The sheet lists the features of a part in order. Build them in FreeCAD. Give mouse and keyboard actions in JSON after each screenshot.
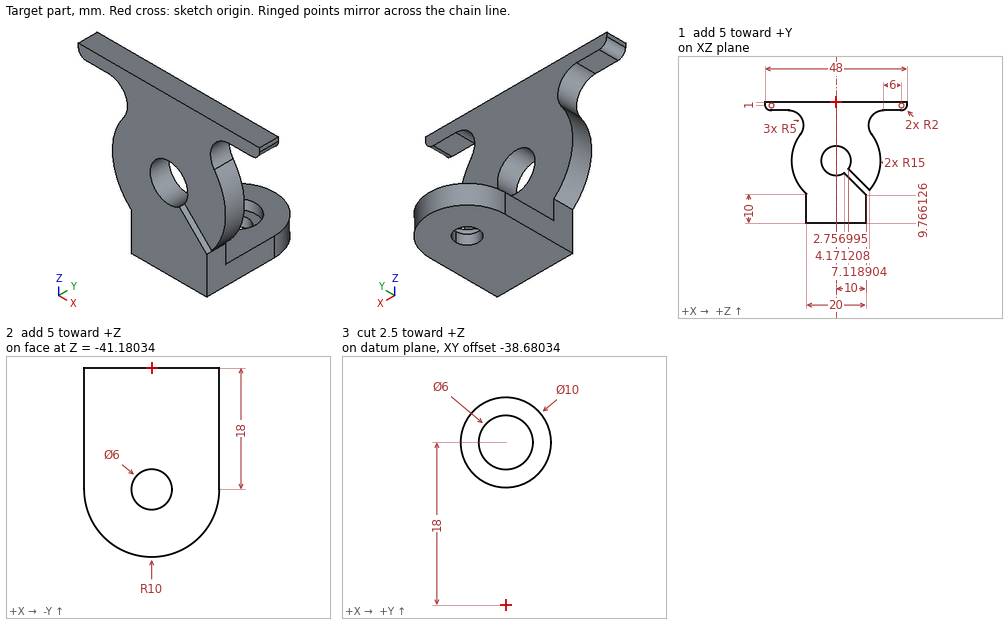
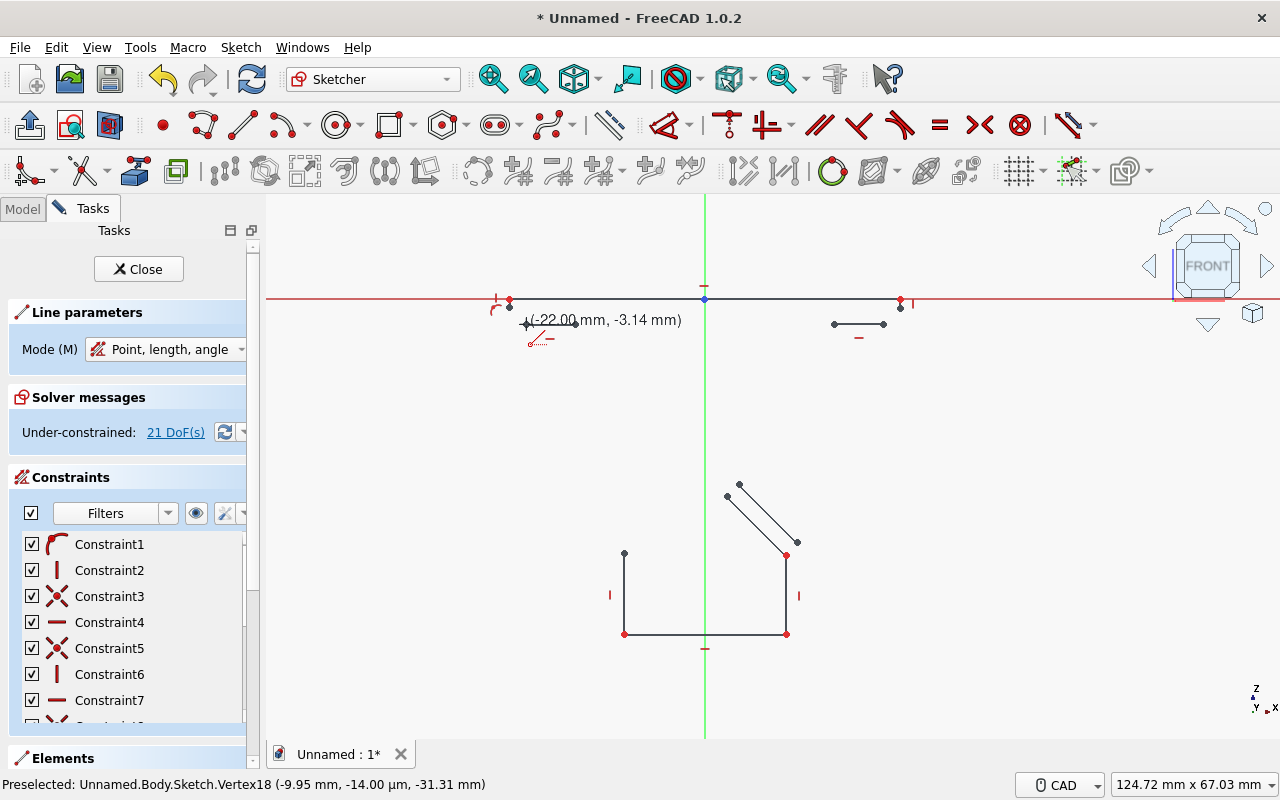
{"action": "key", "text": "g 3 a"}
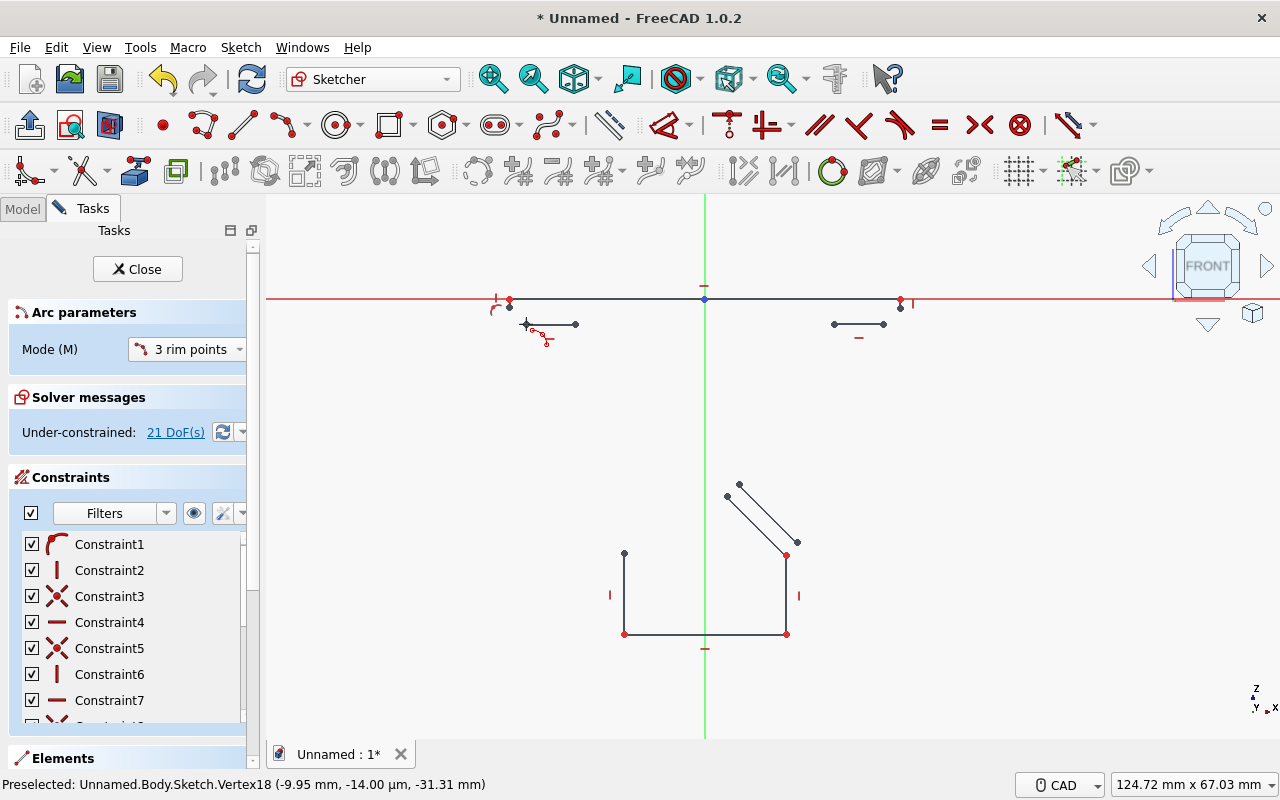
{"action": "scroll", "coordinate": [900, 308], "scroll_direction": "up", "scroll_amount": 7}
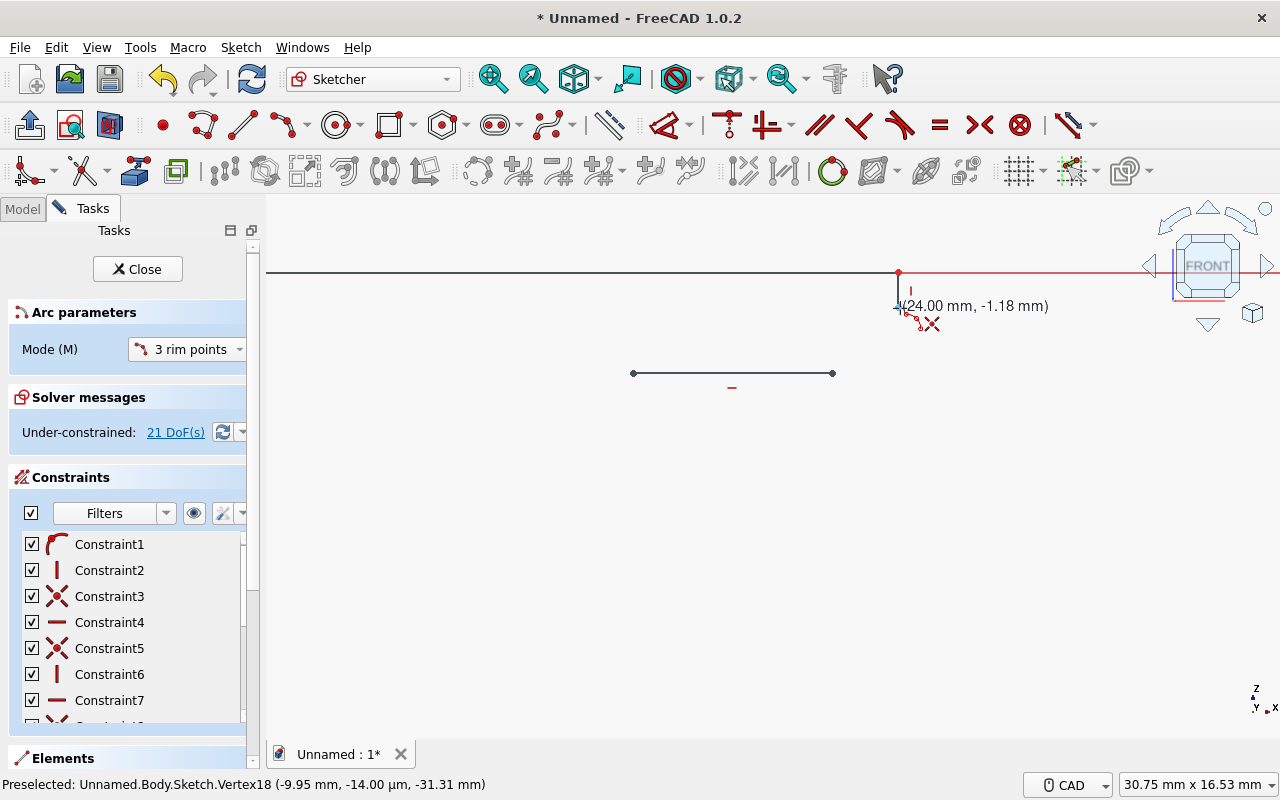
{"action": "left_click", "coordinate": [898, 308]}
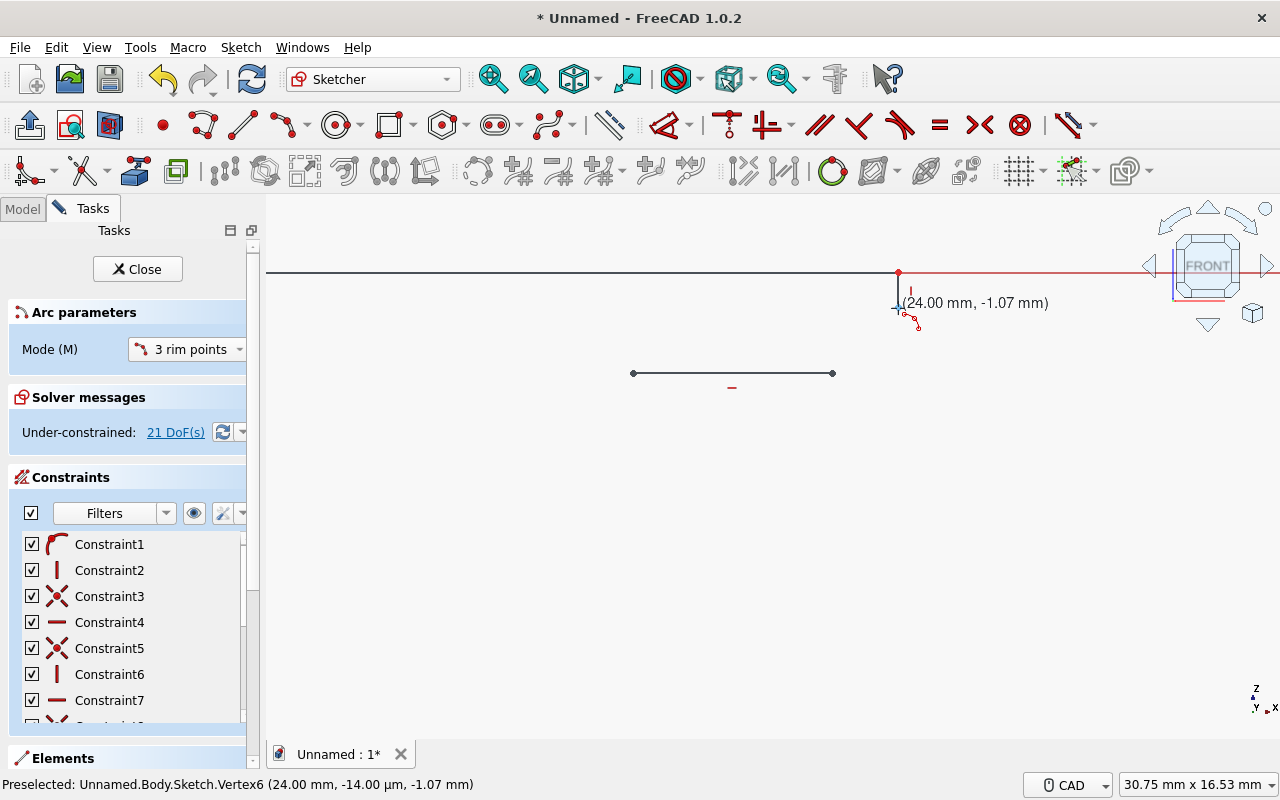
{"action": "scroll", "coordinate": [900, 308], "scroll_direction": "down", "scroll_amount": 7}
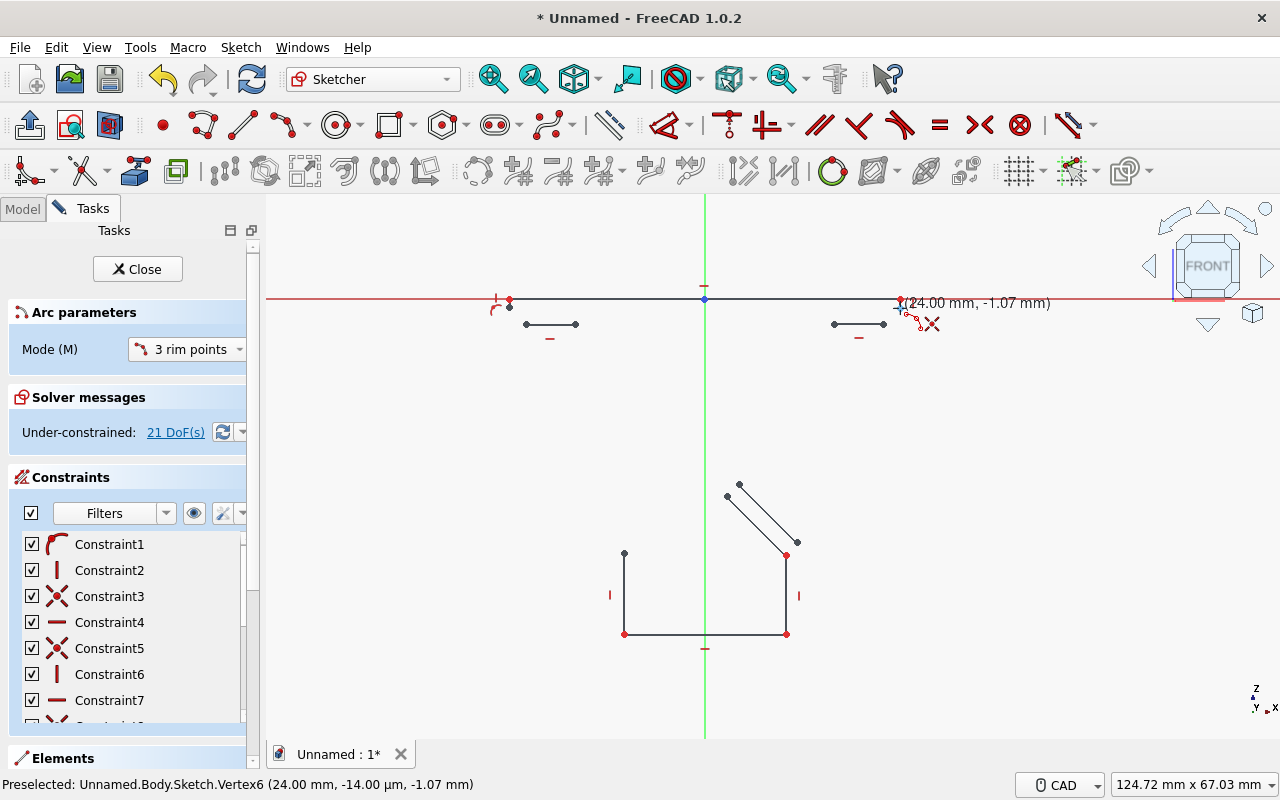
{"action": "left_click", "coordinate": [884, 324]}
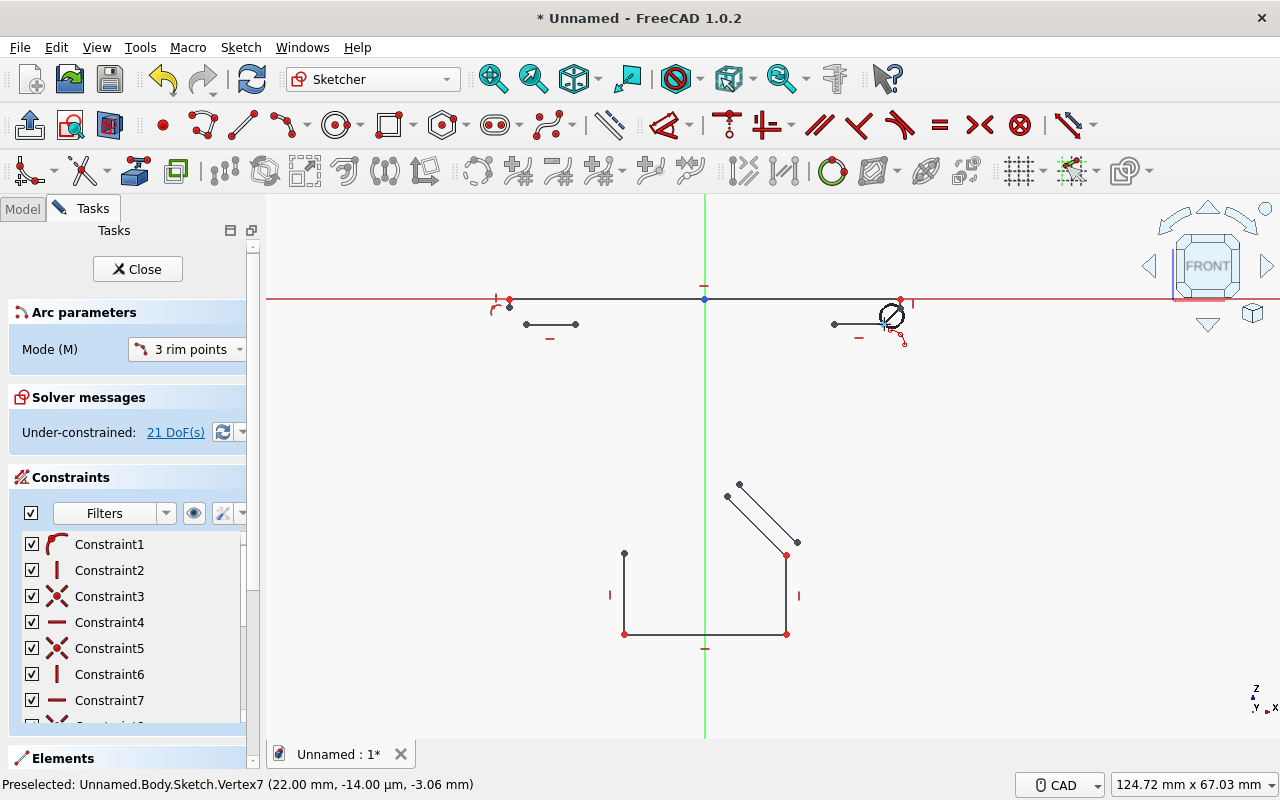
{"action": "scroll", "coordinate": [895, 319], "scroll_direction": "up", "scroll_amount": 7}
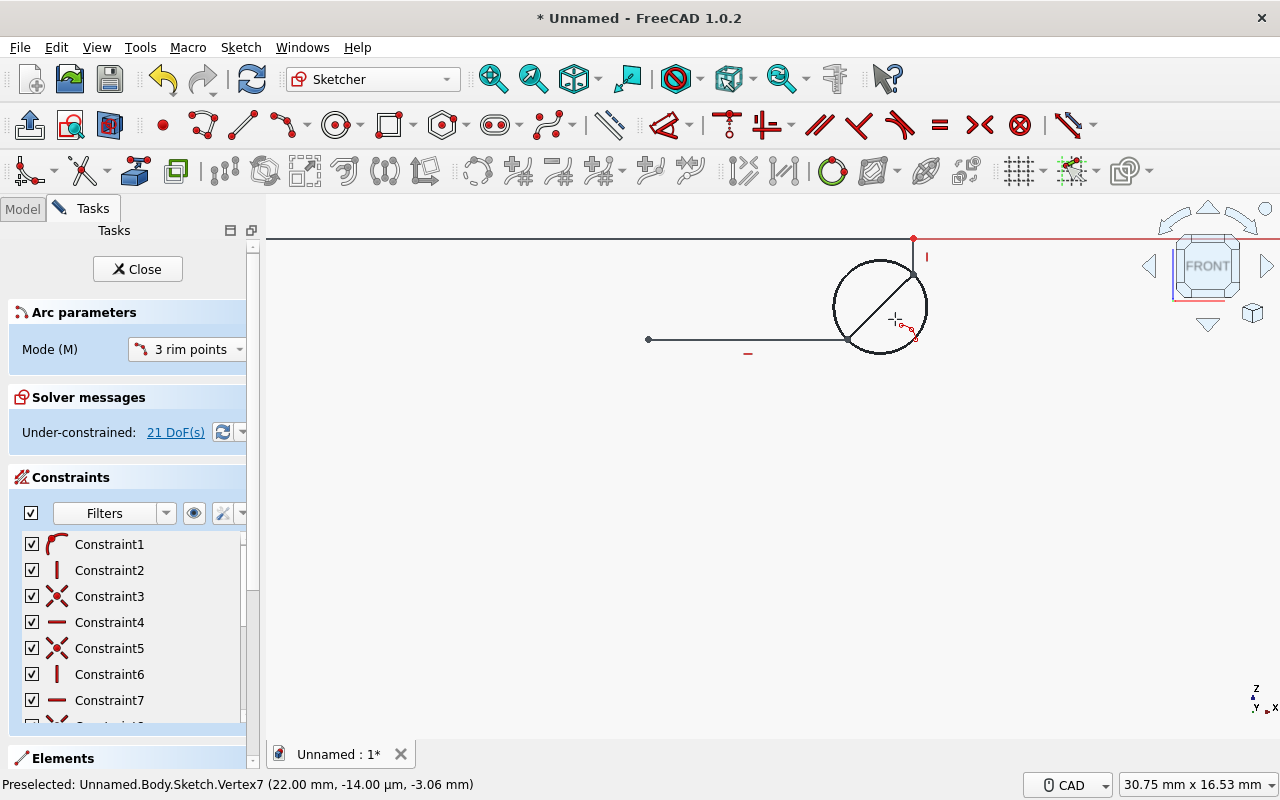
{"action": "left_click", "coordinate": [894, 319]}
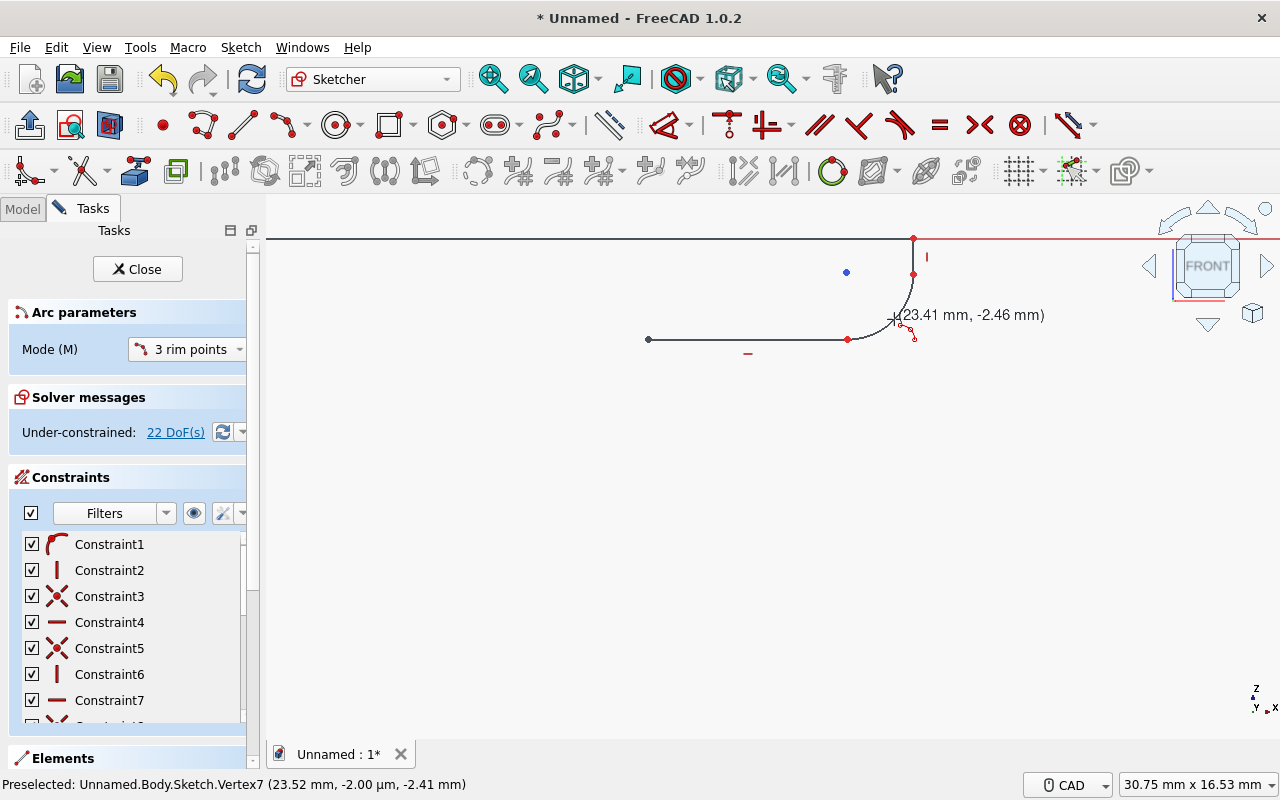
{"action": "scroll", "coordinate": [895, 319], "scroll_direction": "down", "scroll_amount": 7}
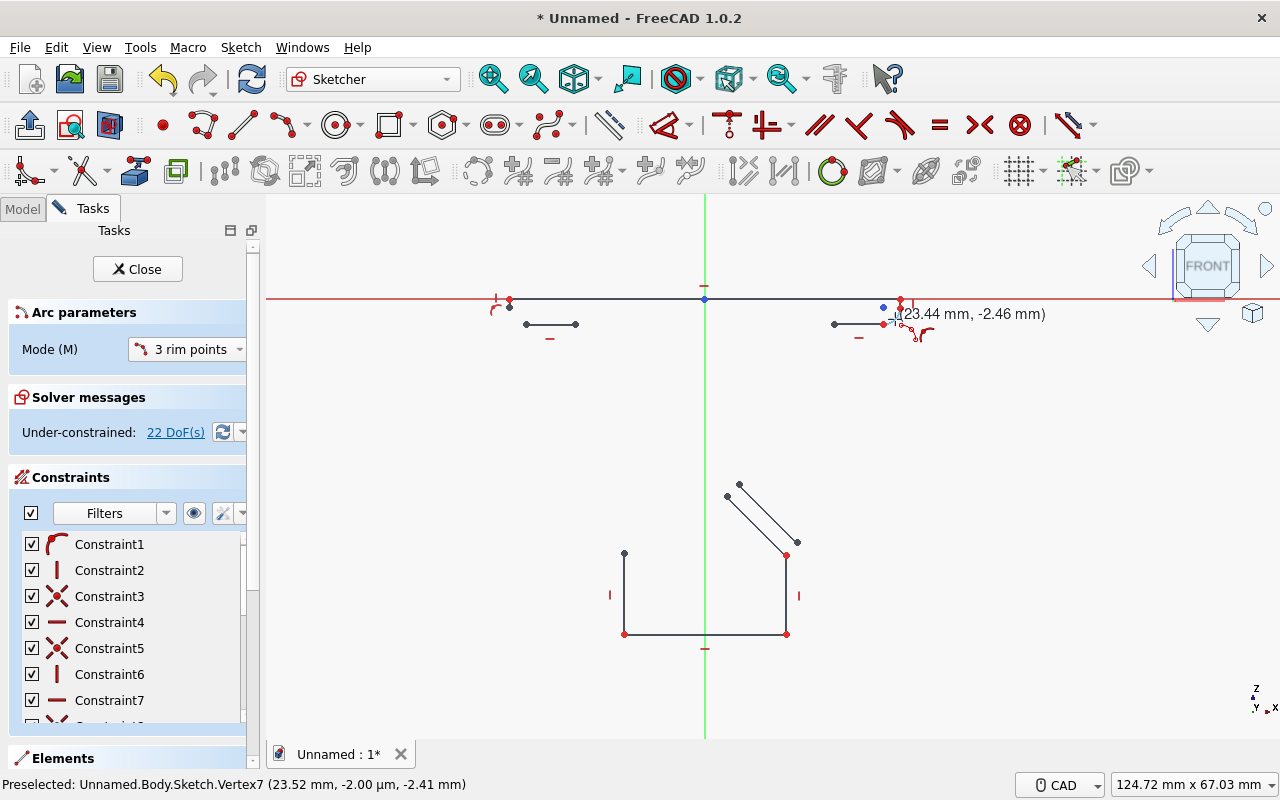
{"action": "left_click", "coordinate": [835, 324]}
{"action": "left_click", "coordinate": [802, 389]}
{"action": "left_click", "coordinate": [799, 346]}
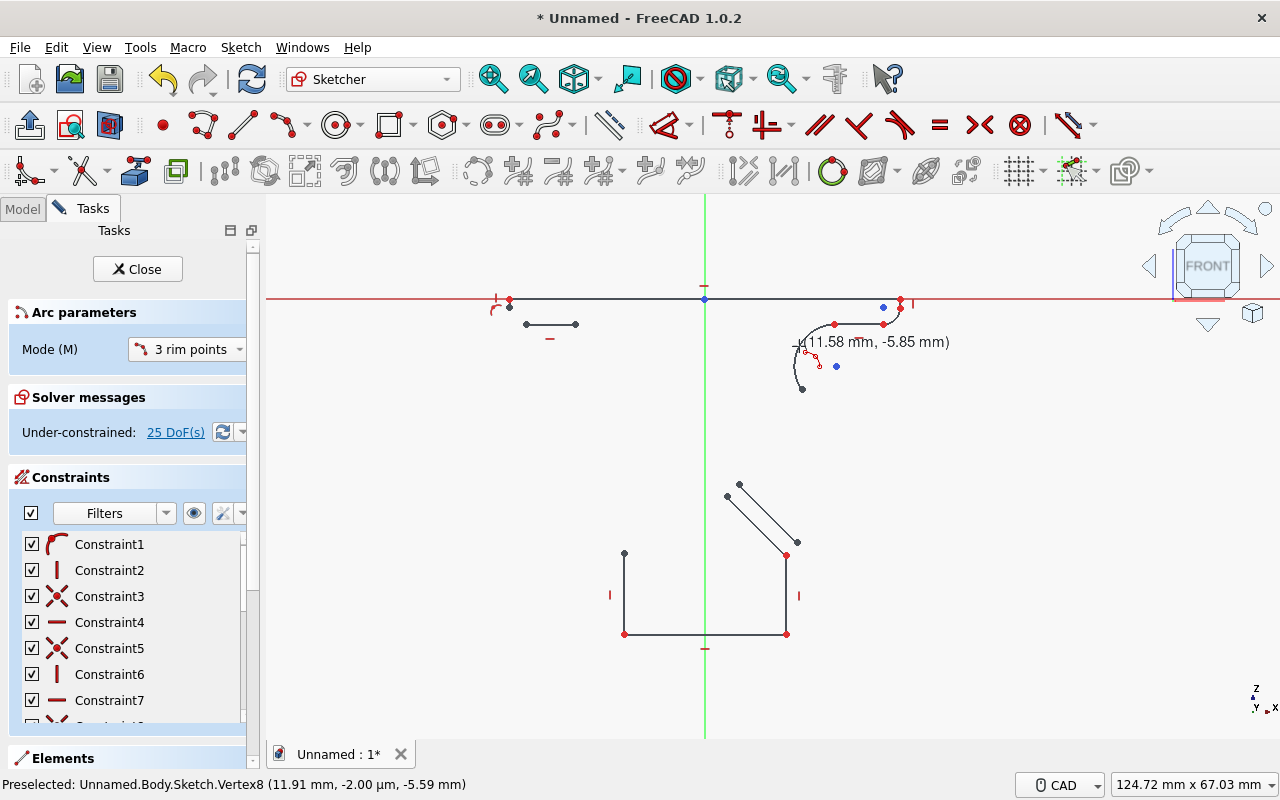
{"action": "left_click", "coordinate": [802, 390]}
{"action": "left_click", "coordinate": [797, 543]}
{"action": "left_click", "coordinate": [827, 467]}